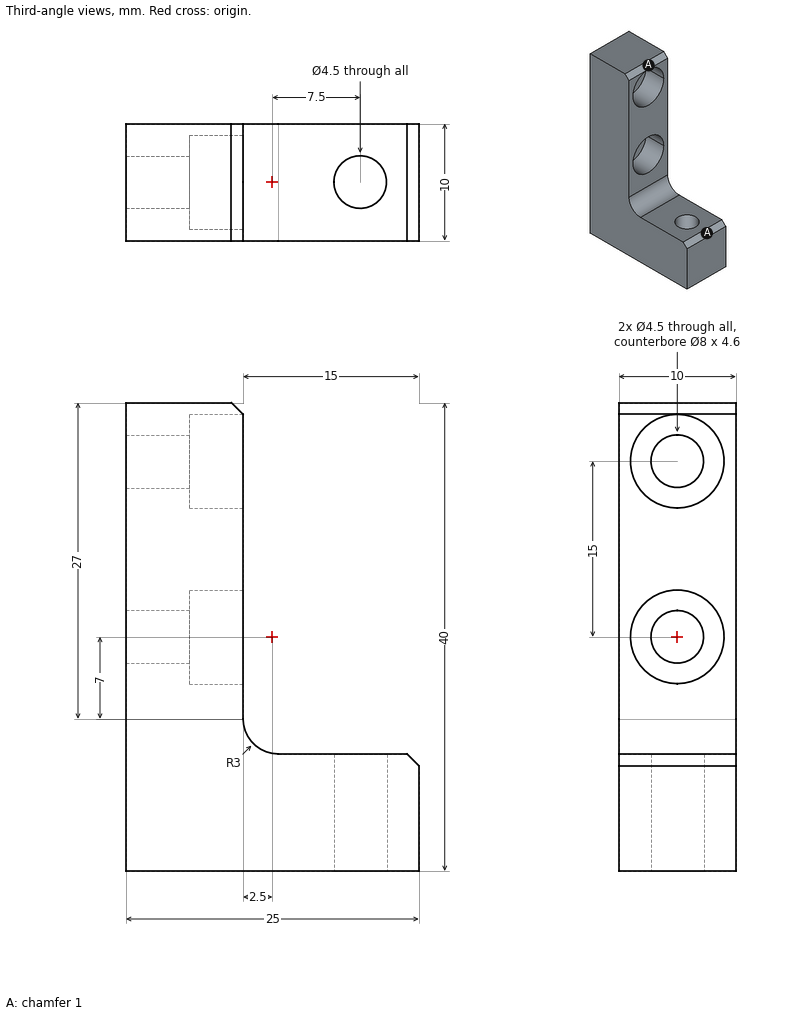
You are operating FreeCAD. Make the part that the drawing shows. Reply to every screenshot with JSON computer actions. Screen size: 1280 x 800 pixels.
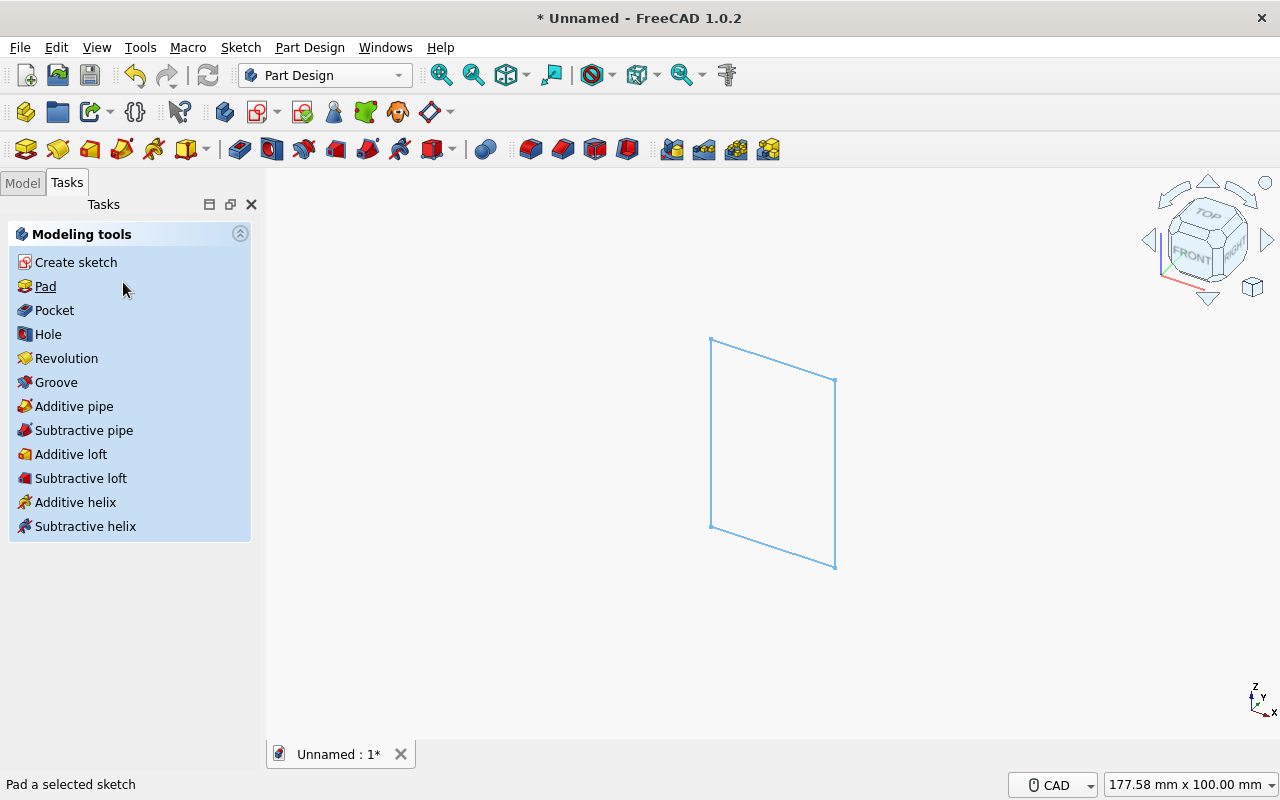
{"action": "left_click", "coordinate": [26, 150]}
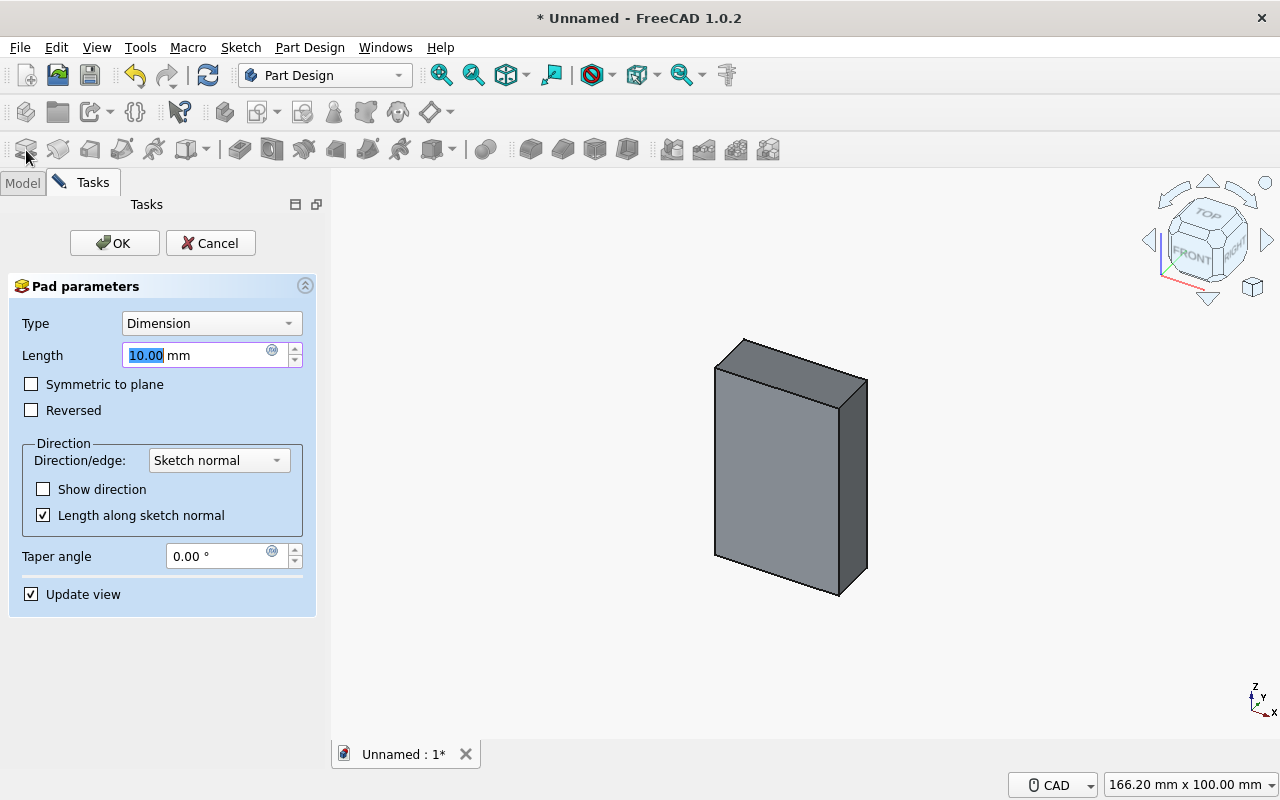
{"action": "type", "text": "10"}
{"action": "key", "text": "Tab"}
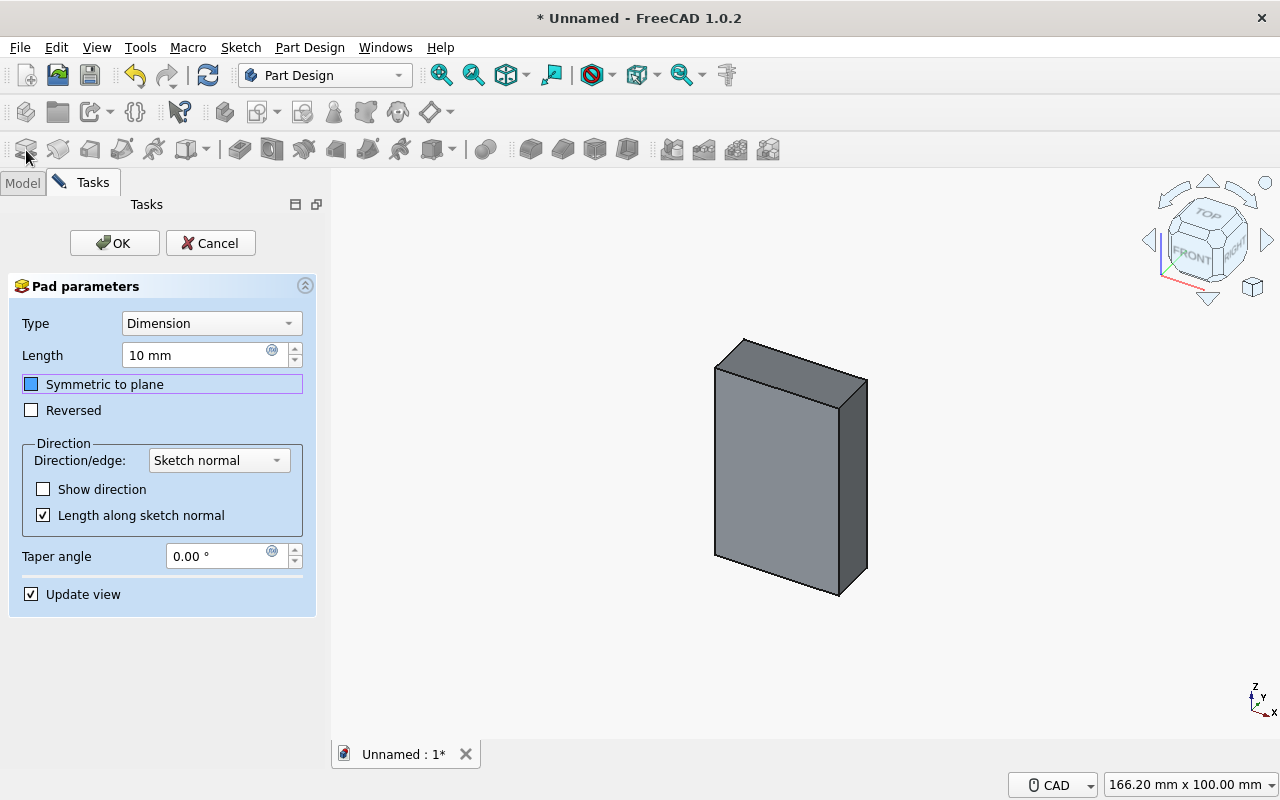
{"action": "left_click", "coordinate": [30, 384]}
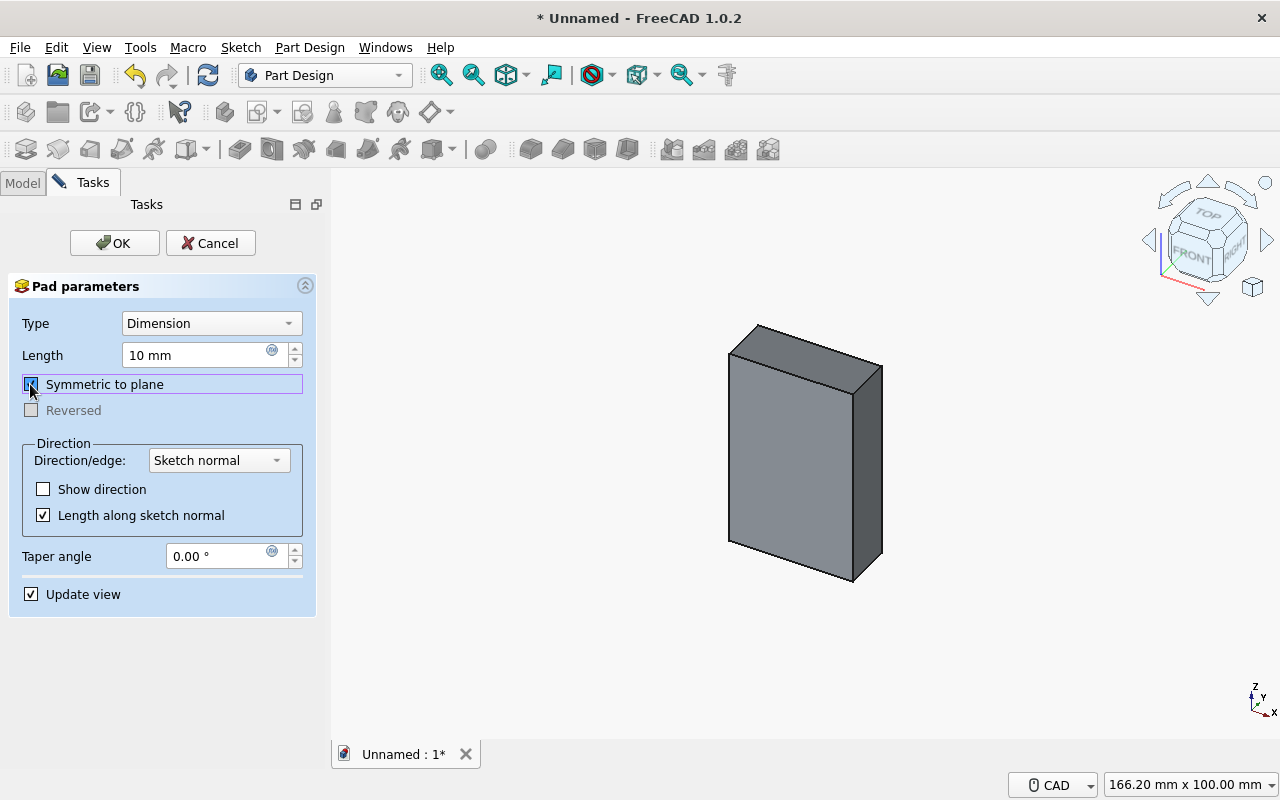
{"action": "left_click", "coordinate": [115, 243]}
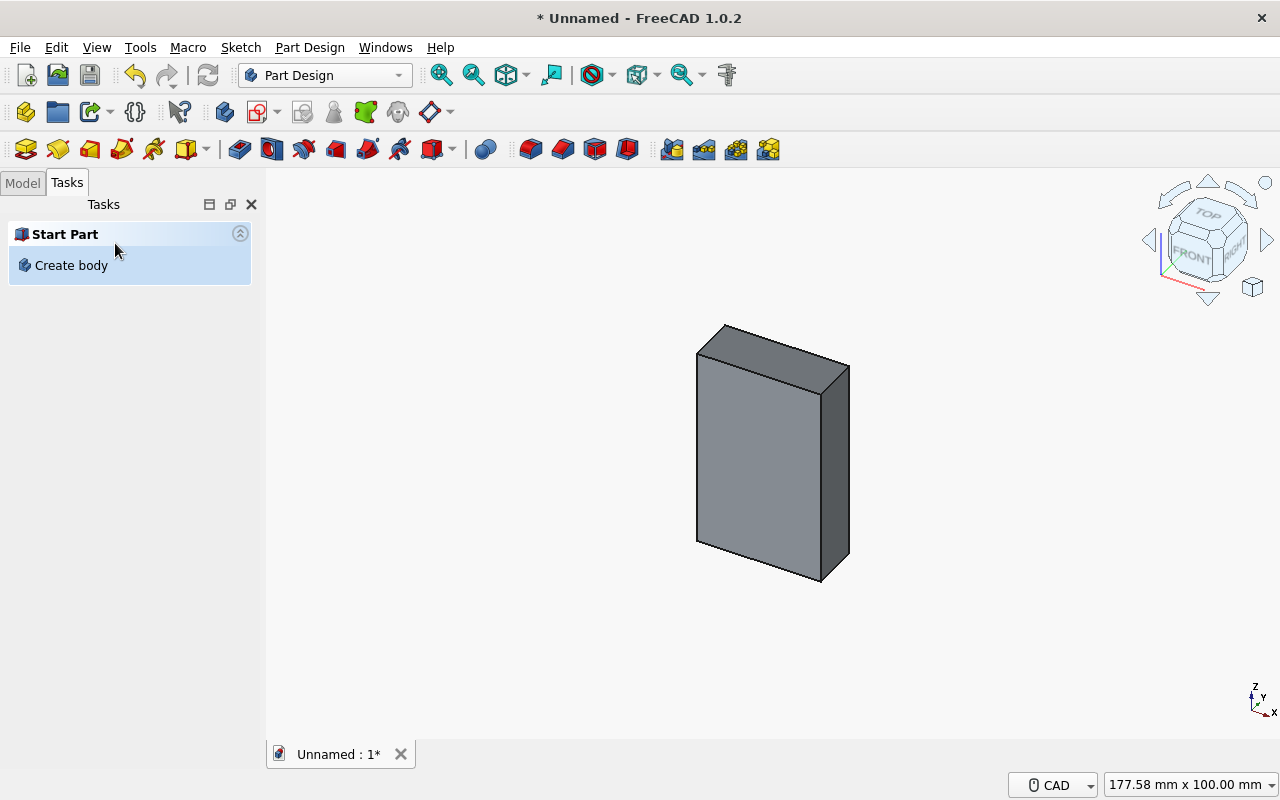
{"action": "key", "text": "4"}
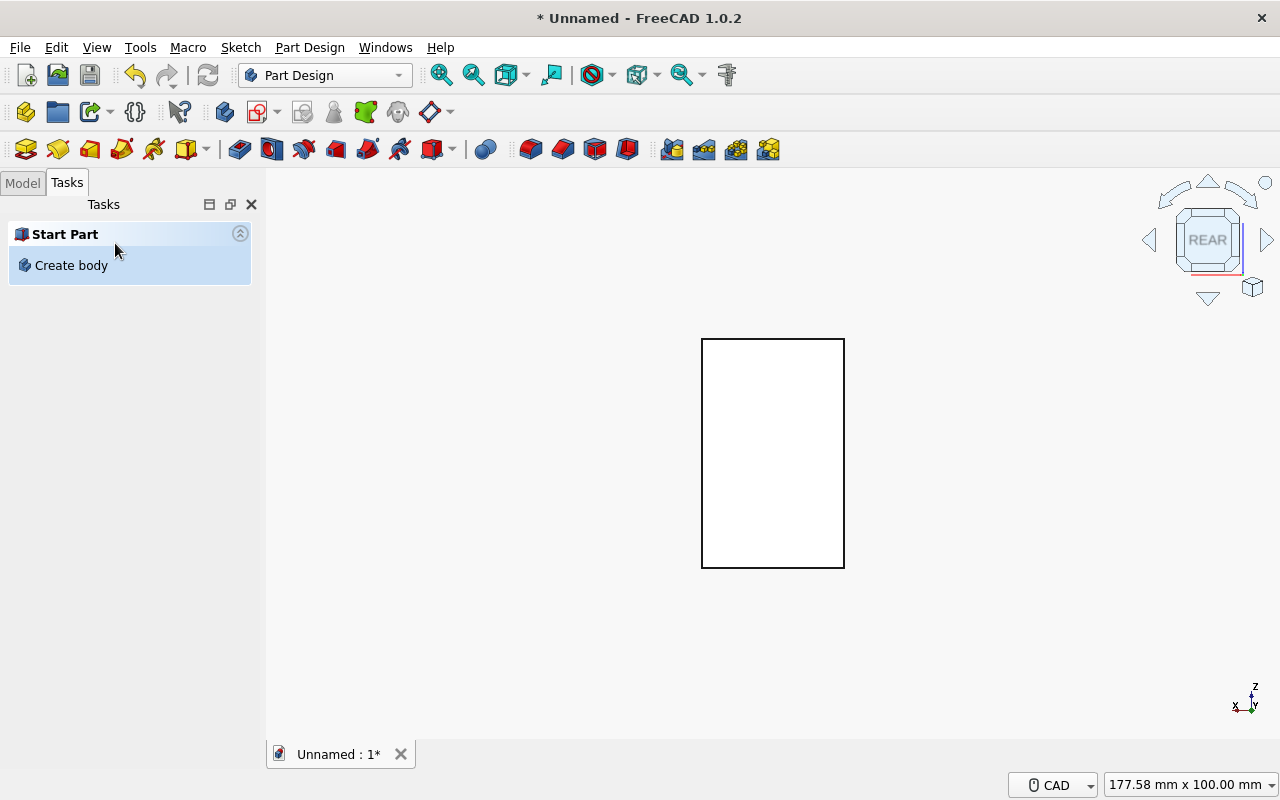
{"action": "left_click", "coordinate": [442, 76]}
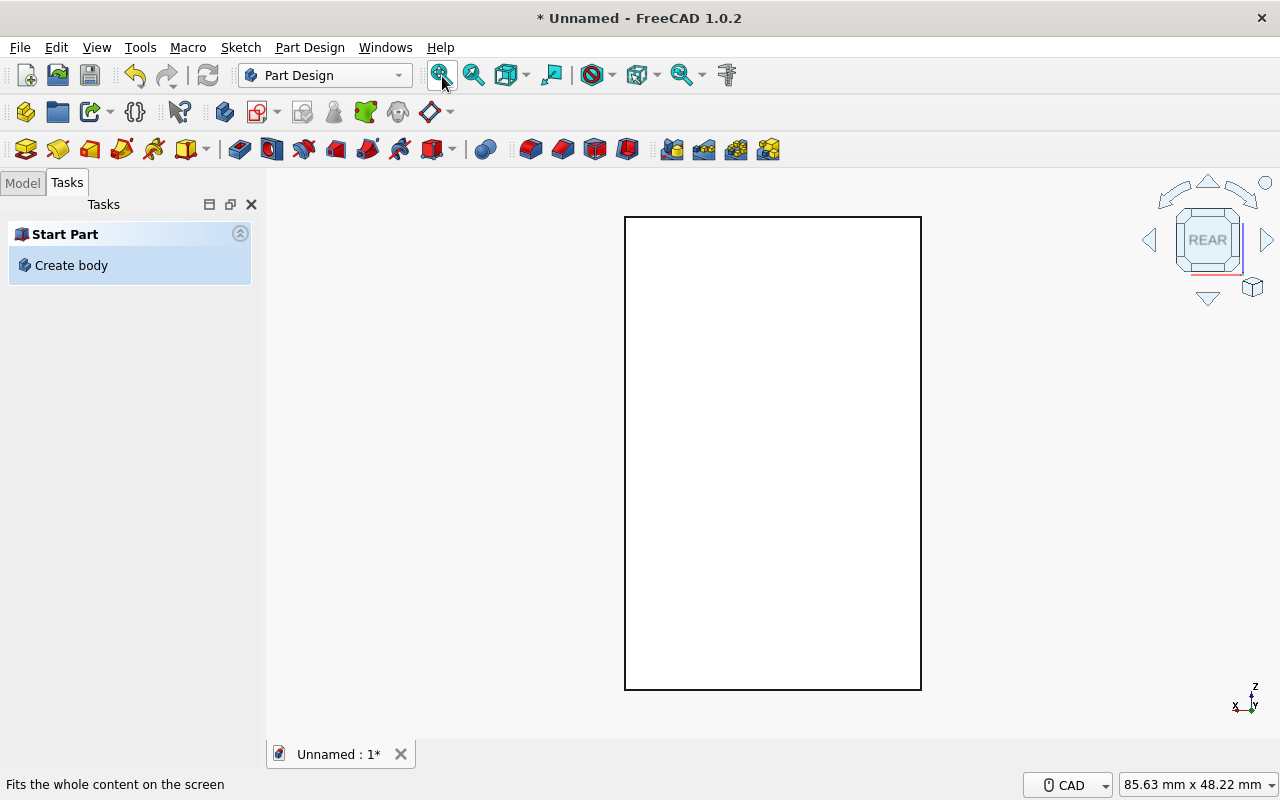
{"action": "left_click", "coordinate": [773, 385]}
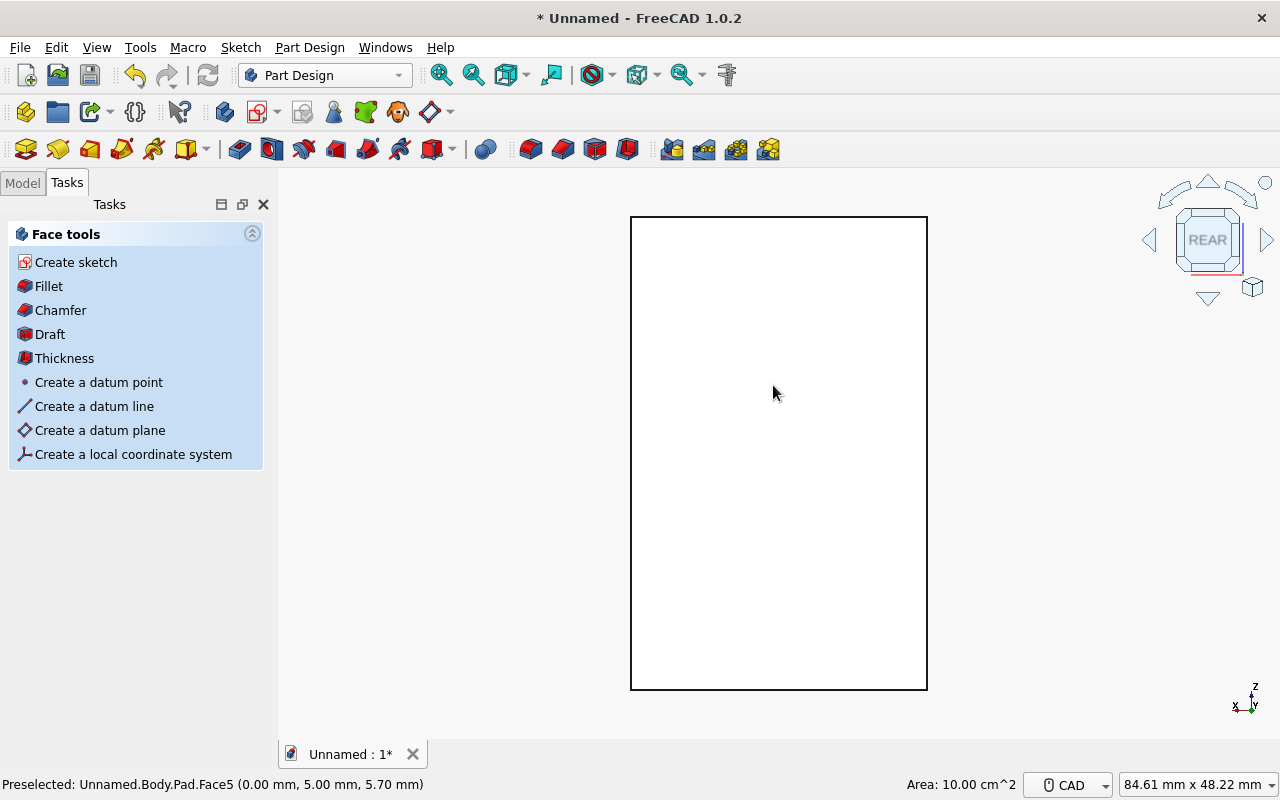
{"action": "left_click", "coordinate": [258, 112]}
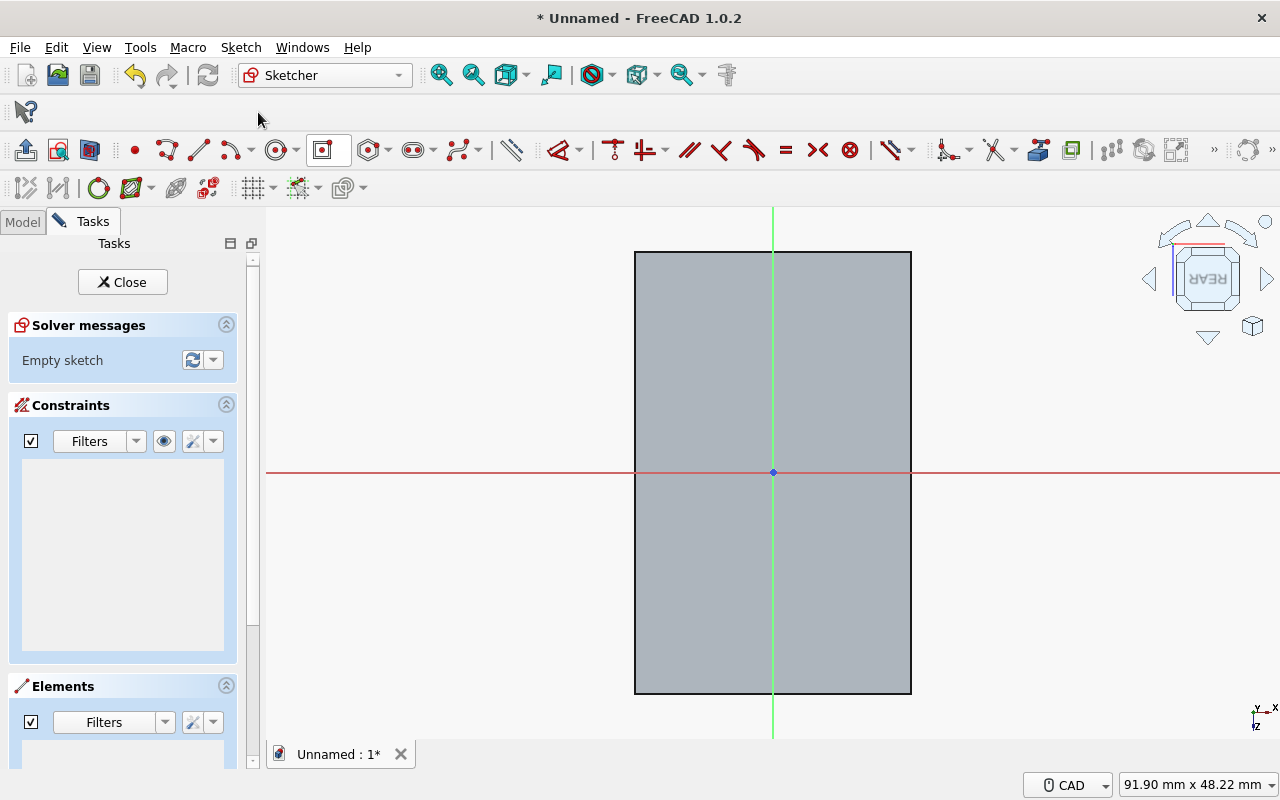
{"action": "scroll", "coordinate": [294, 235], "scroll_direction": "down", "scroll_amount": 1}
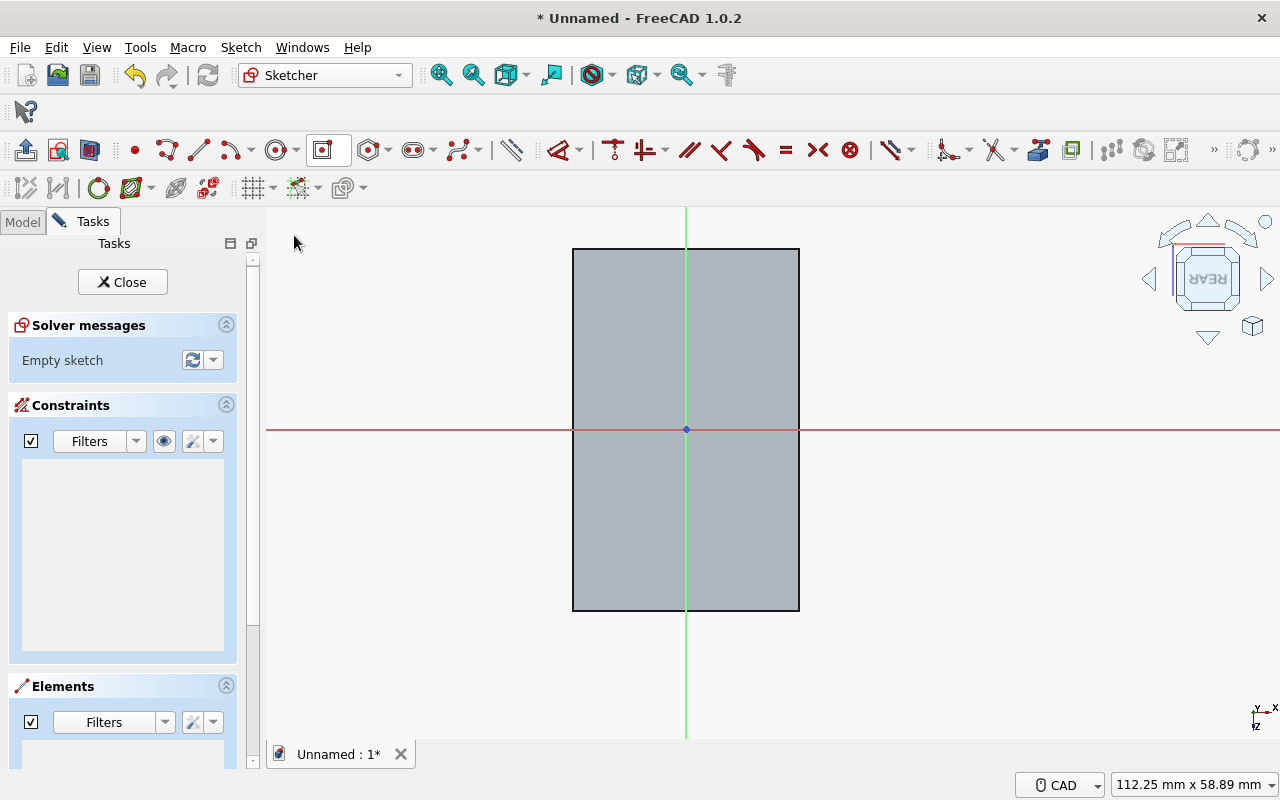
{"action": "left_click", "coordinate": [168, 150]}